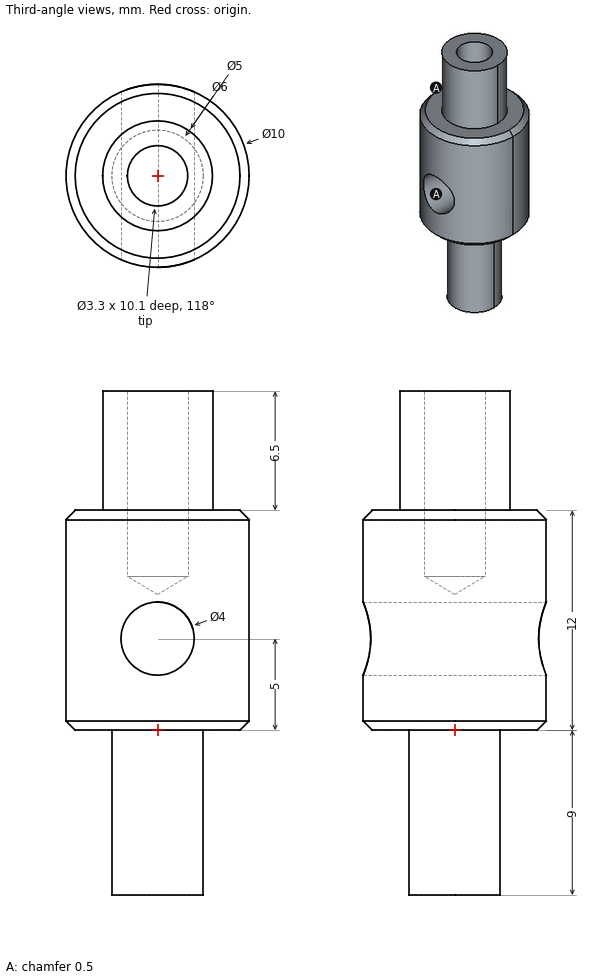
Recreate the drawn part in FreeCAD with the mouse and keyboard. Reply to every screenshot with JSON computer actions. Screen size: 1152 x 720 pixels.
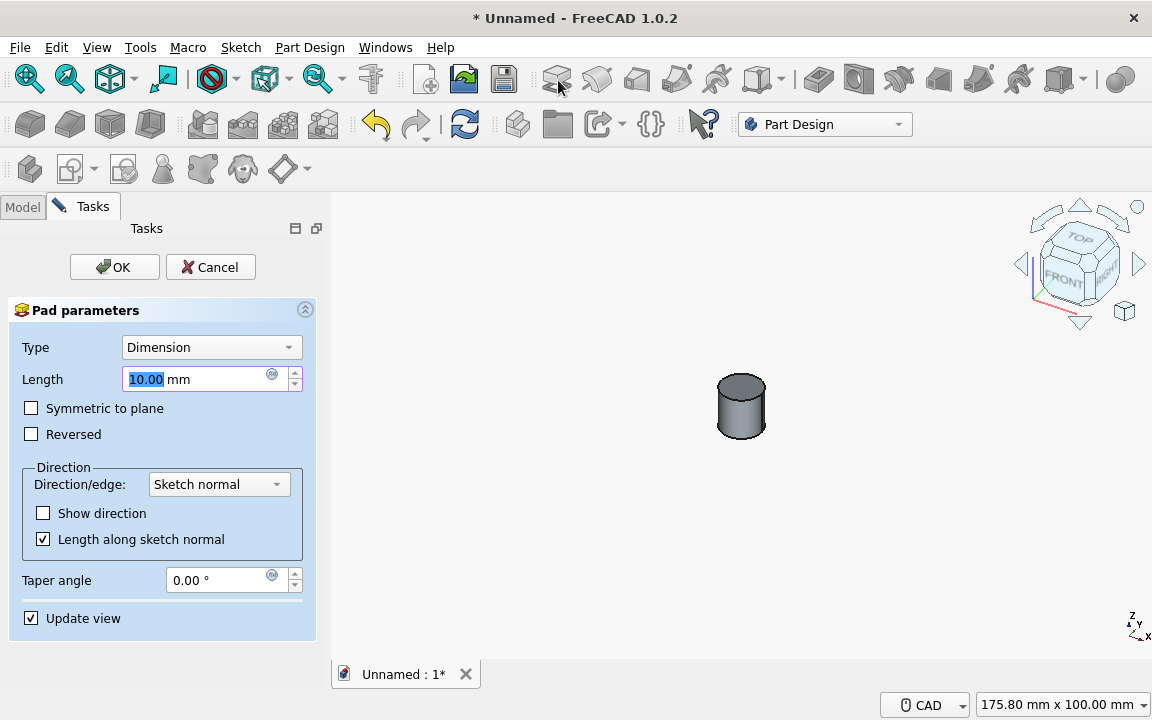
{"action": "type", "text": "12"}
{"action": "key", "text": "Tab"}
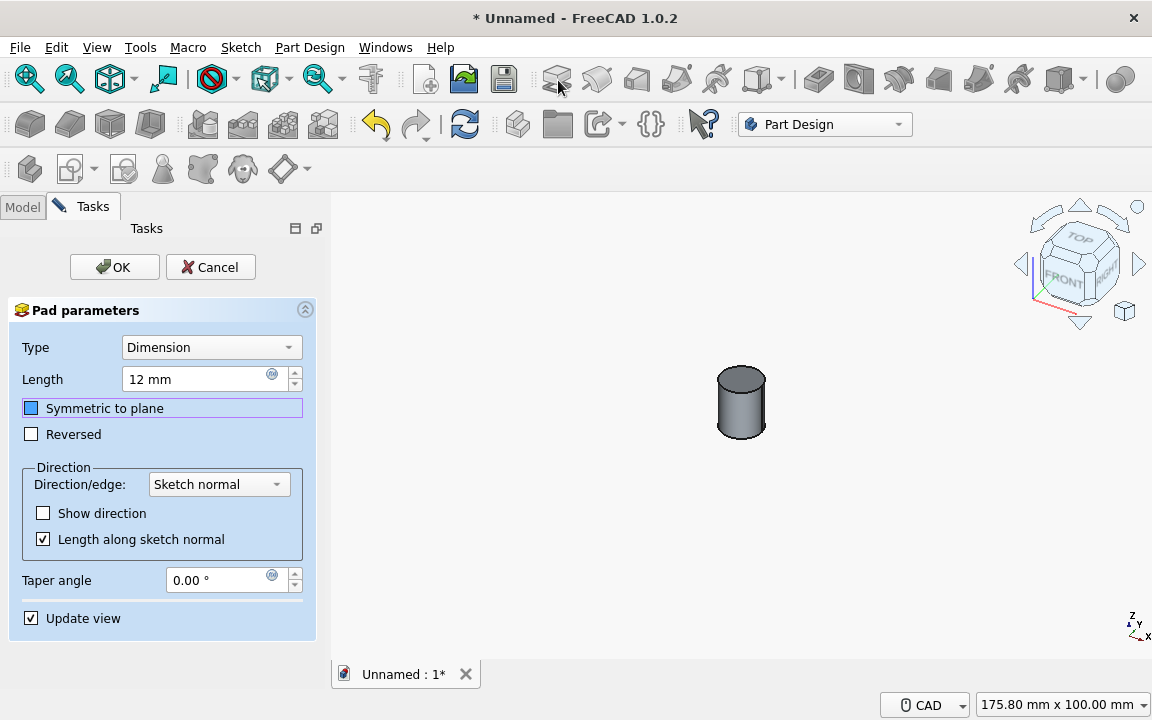
{"action": "left_click", "coordinate": [115, 267]}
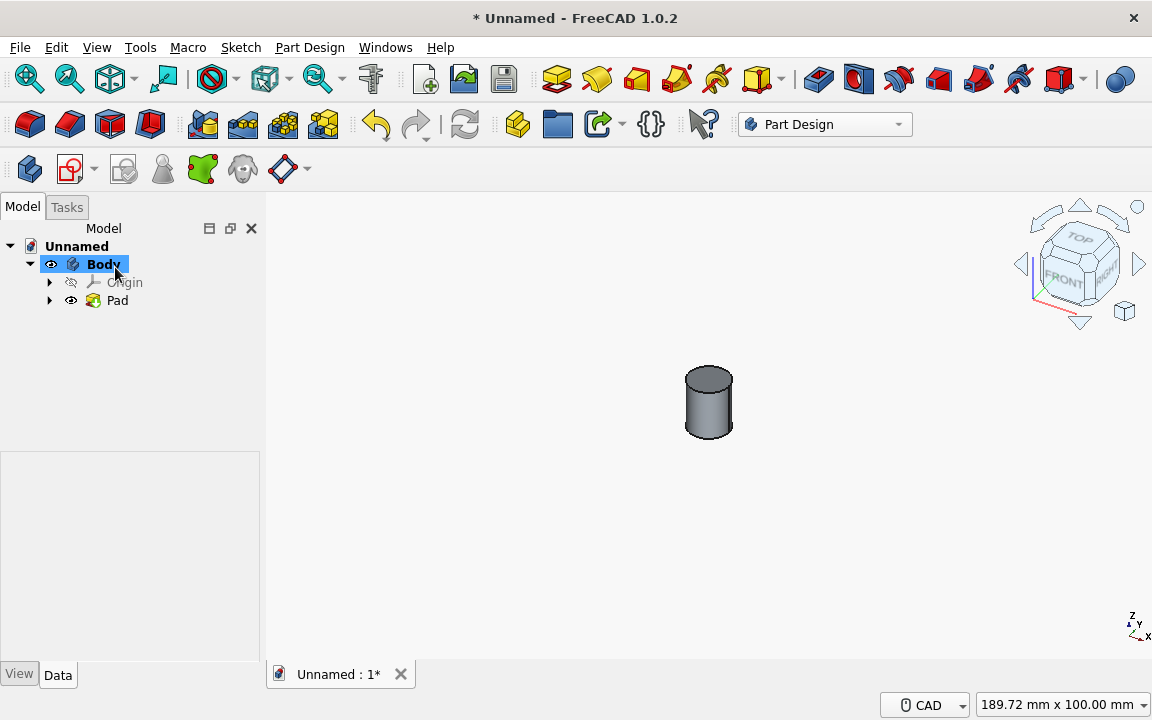
{"action": "key", "text": "v f"}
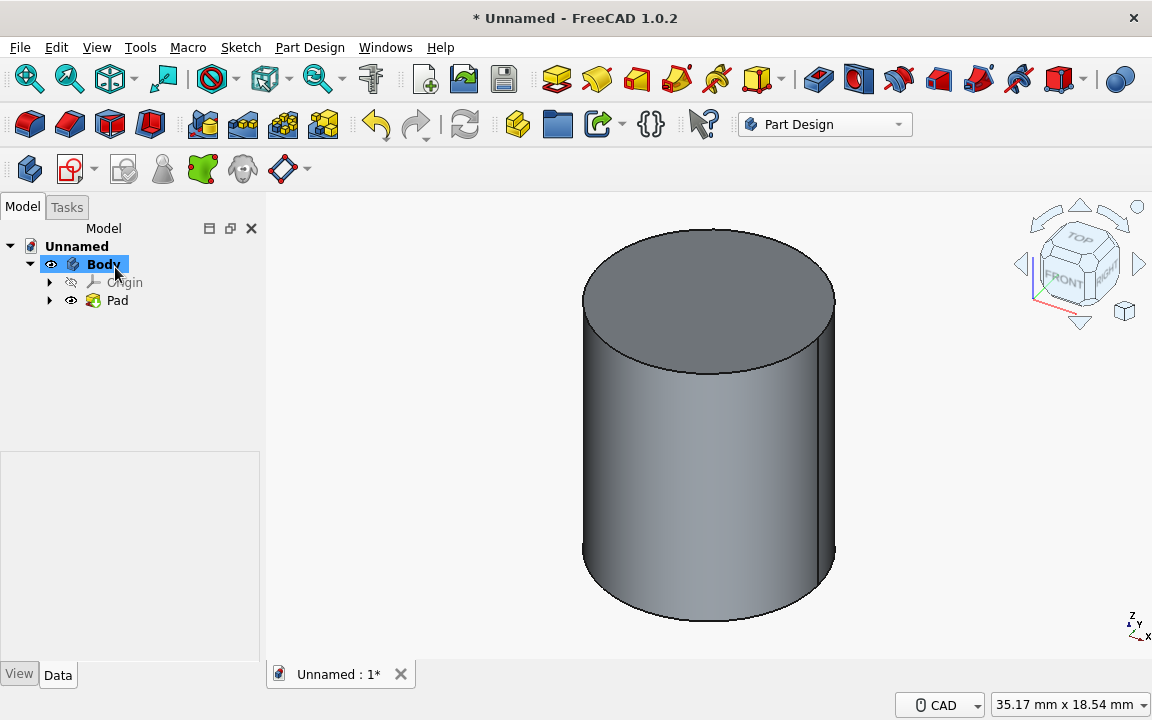
{"action": "left_click", "coordinate": [709, 301]}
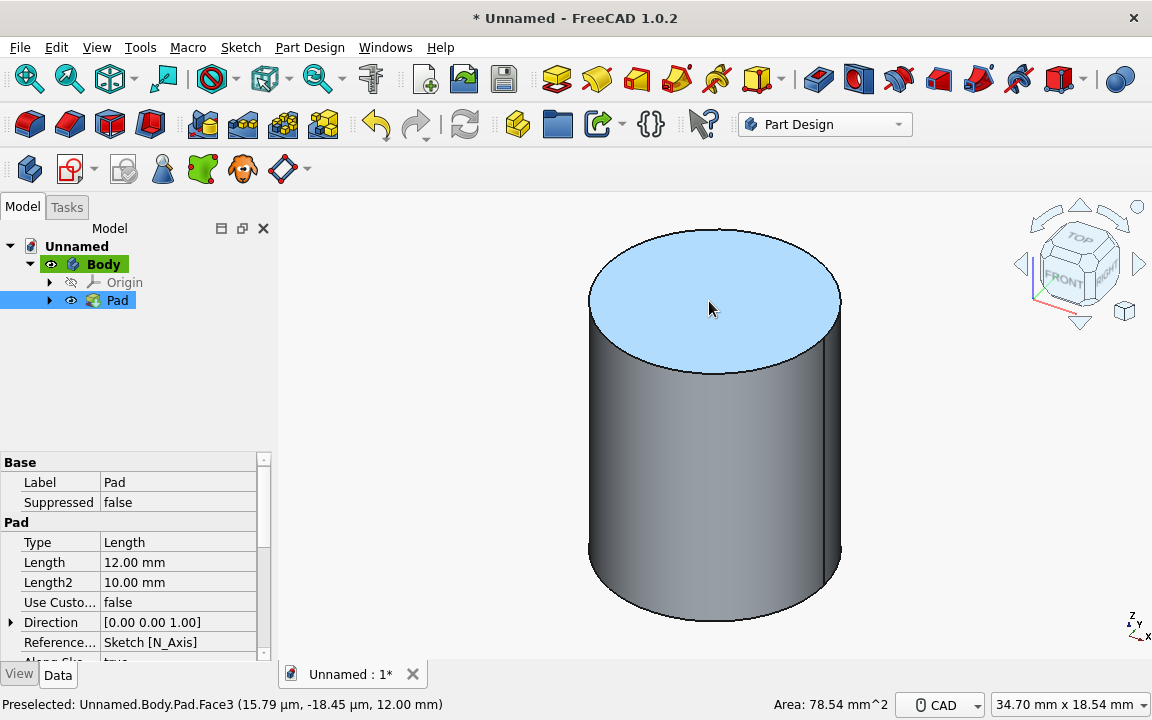
{"action": "left_click", "coordinate": [70, 170]}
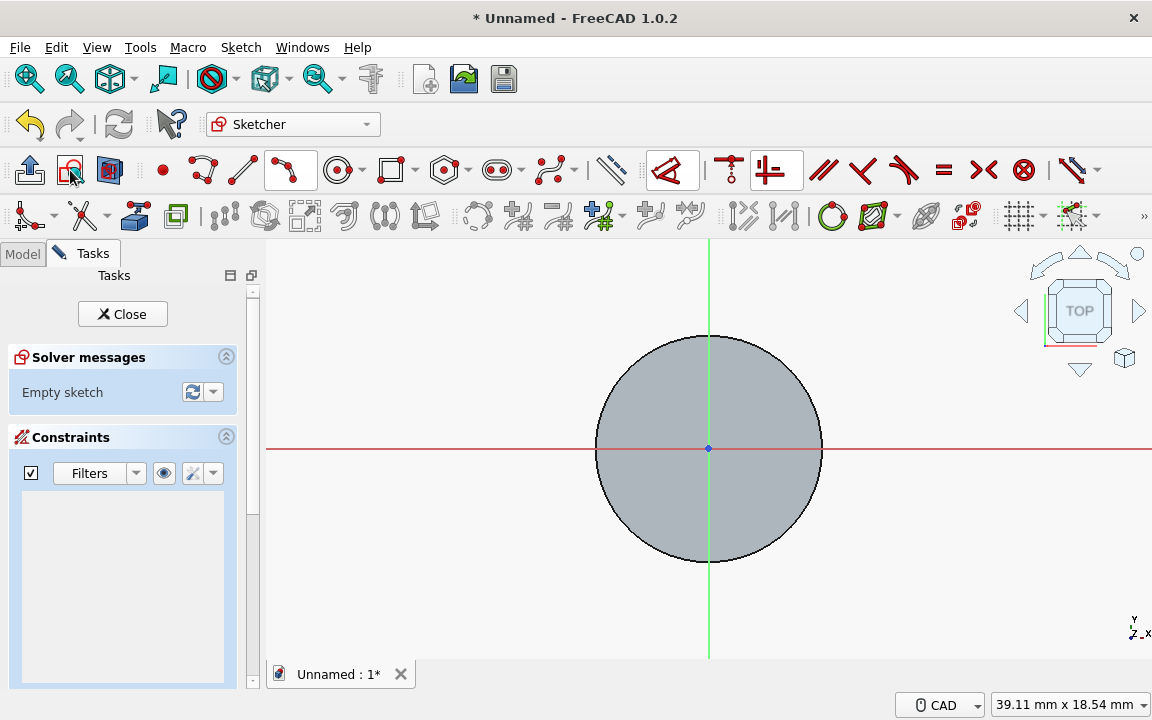
{"action": "scroll", "coordinate": [792, 449], "scroll_direction": "up", "scroll_amount": 3}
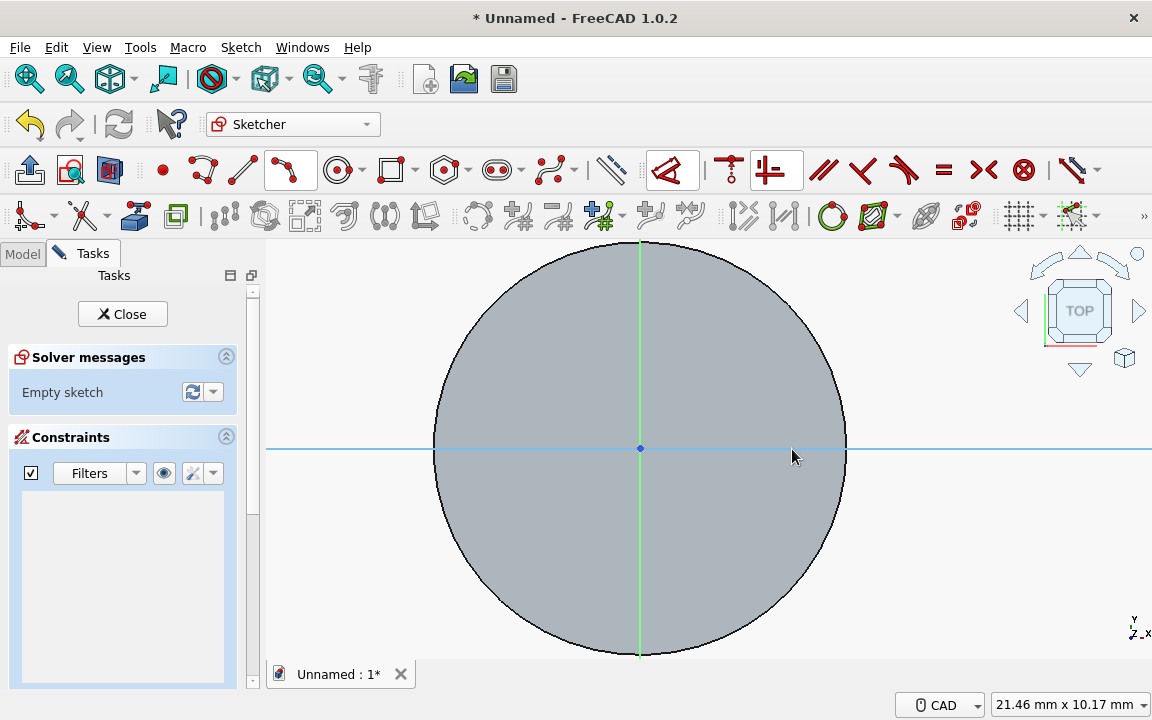
{"action": "left_click", "coordinate": [338, 170]}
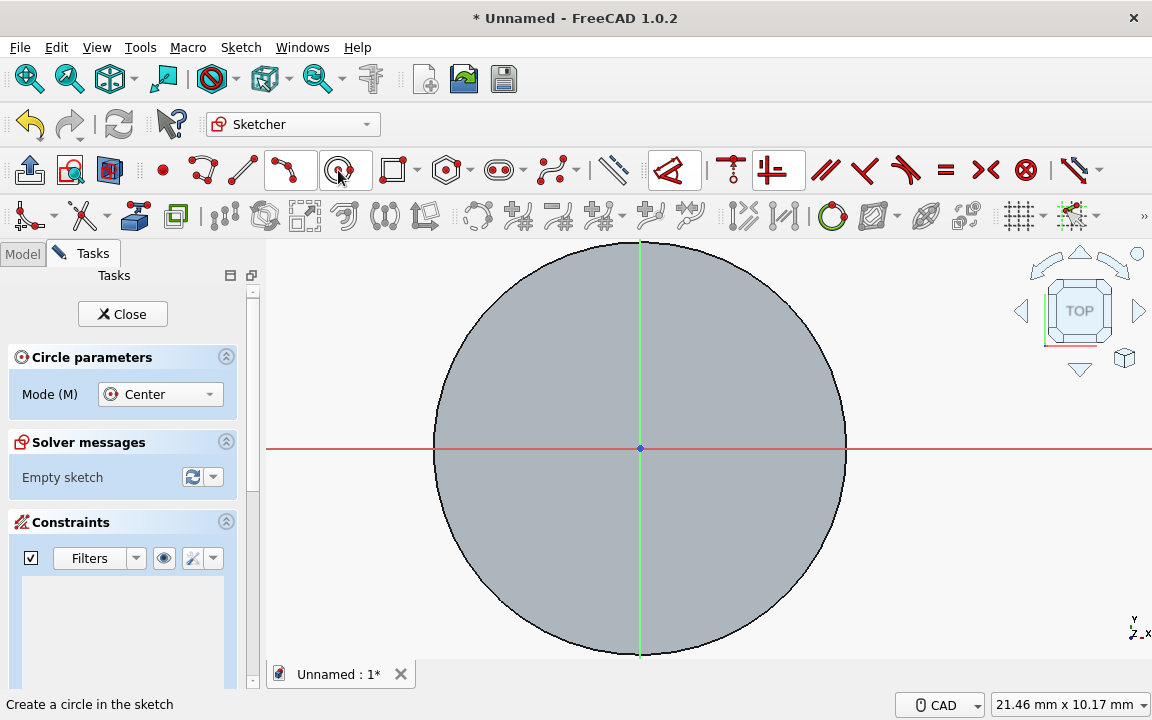
{"action": "left_click", "coordinate": [640, 449]}
{"action": "left_click", "coordinate": [728, 361]}
{"action": "key", "text": "Escape"}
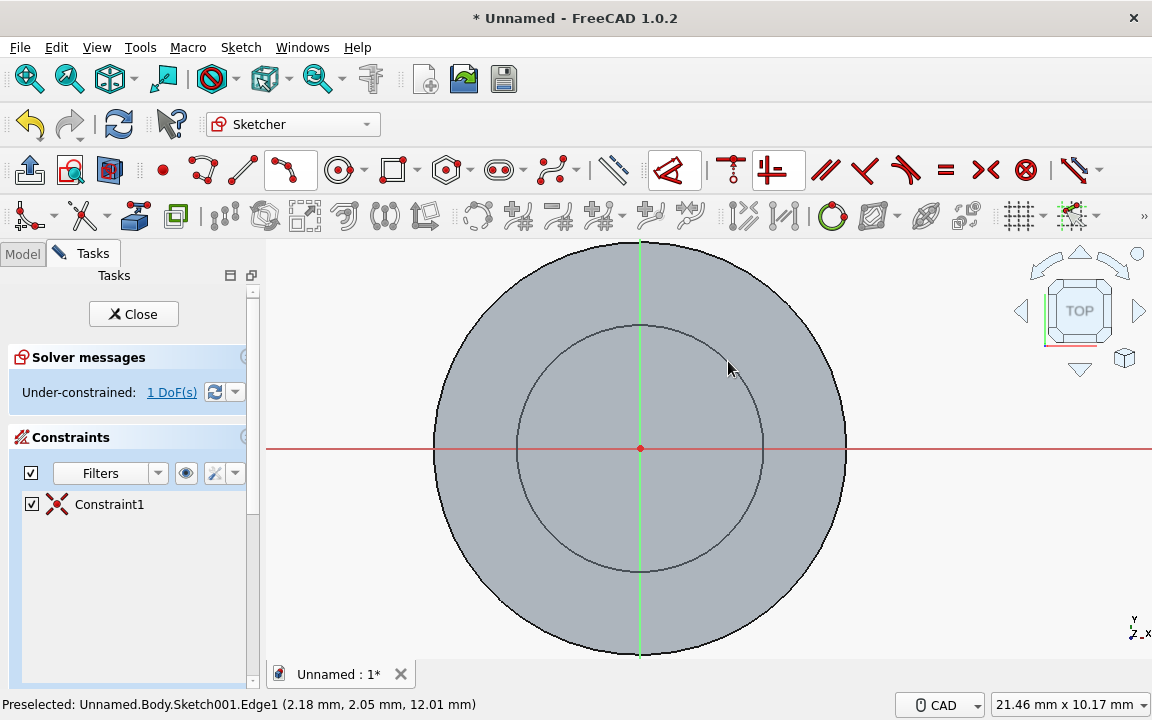
{"action": "left_click", "coordinate": [668, 170]}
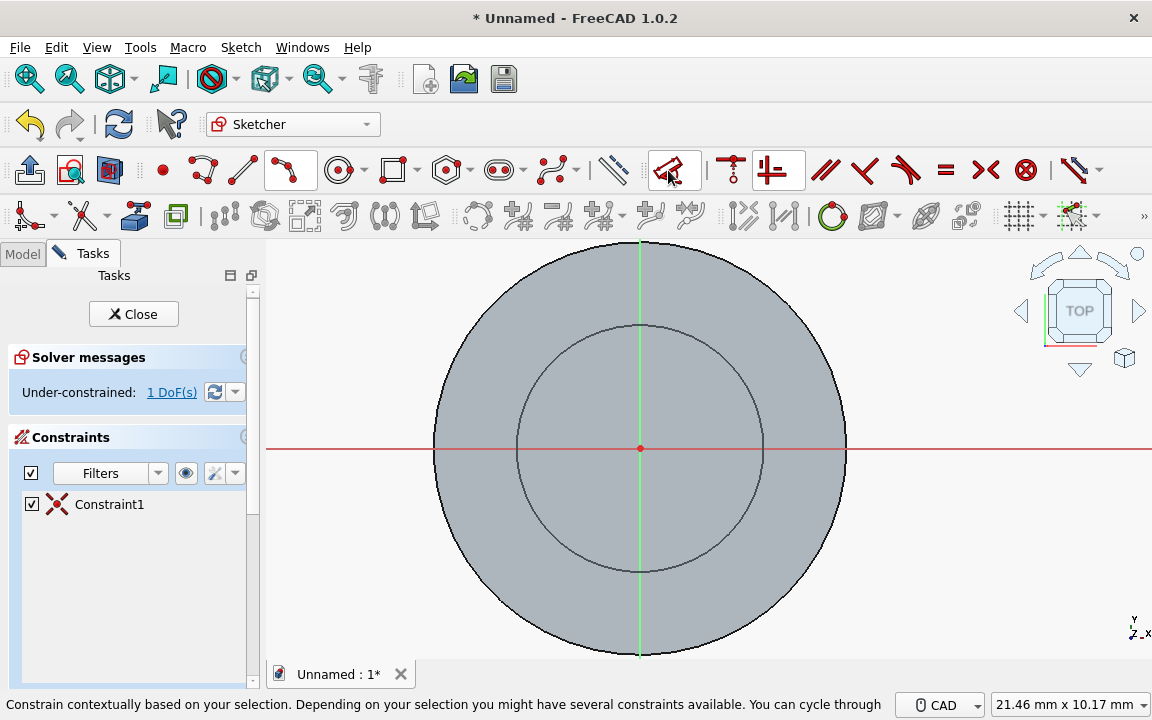
{"action": "left_click", "coordinate": [727, 361]}
{"action": "left_click", "coordinate": [750, 338]}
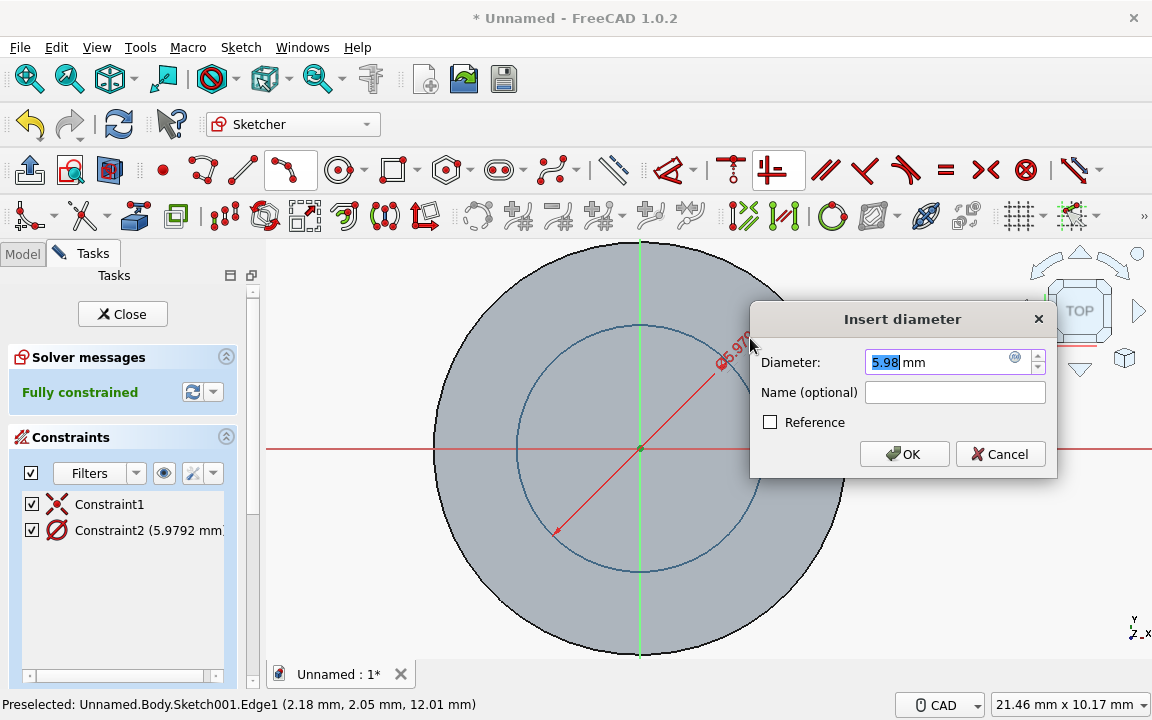
{"action": "type", "text": "6"}
{"action": "key", "text": "Return"}
{"action": "key", "text": "Escape"}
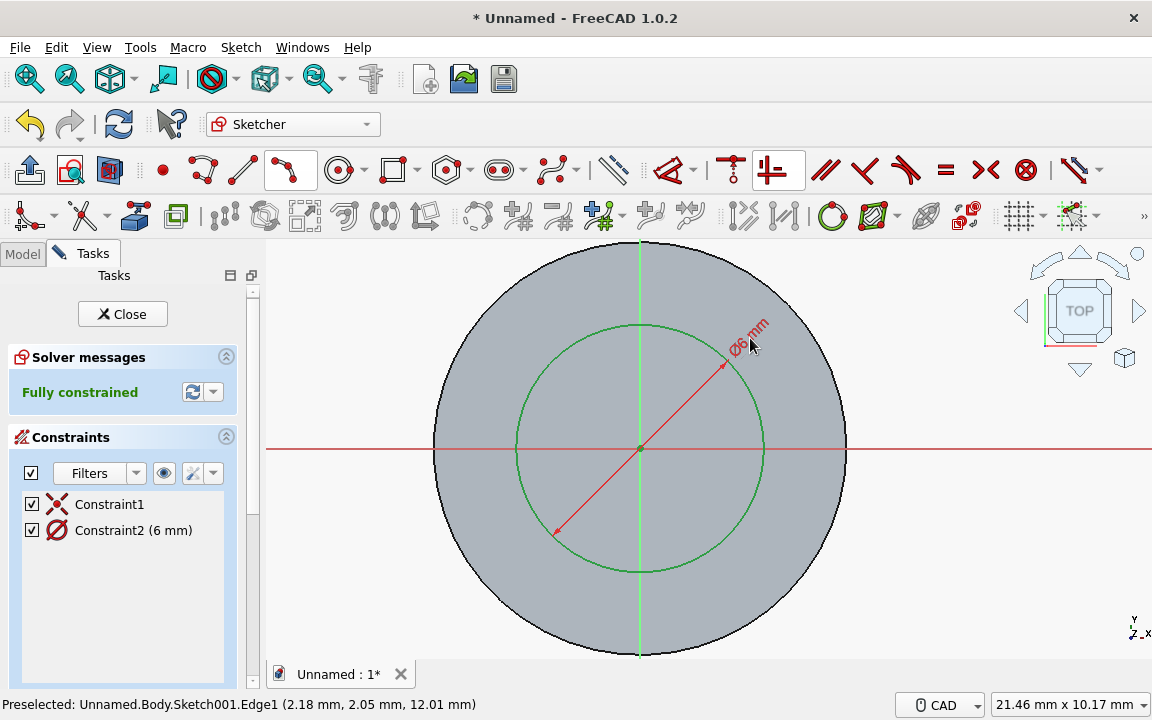
{"action": "left_click", "coordinate": [123, 314]}